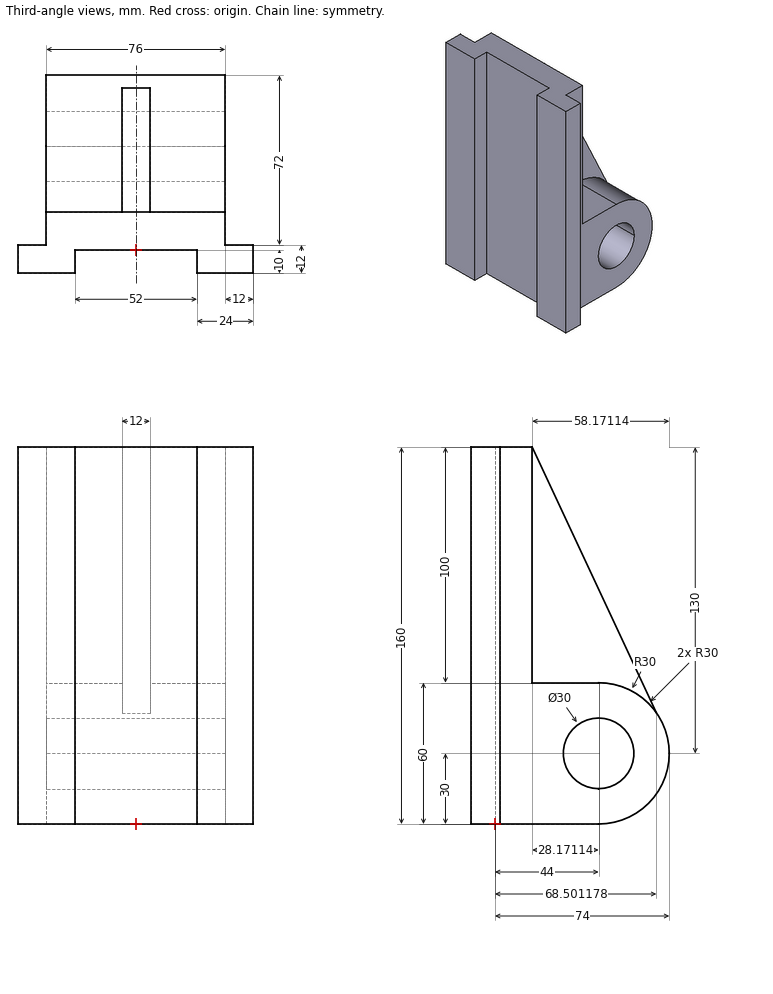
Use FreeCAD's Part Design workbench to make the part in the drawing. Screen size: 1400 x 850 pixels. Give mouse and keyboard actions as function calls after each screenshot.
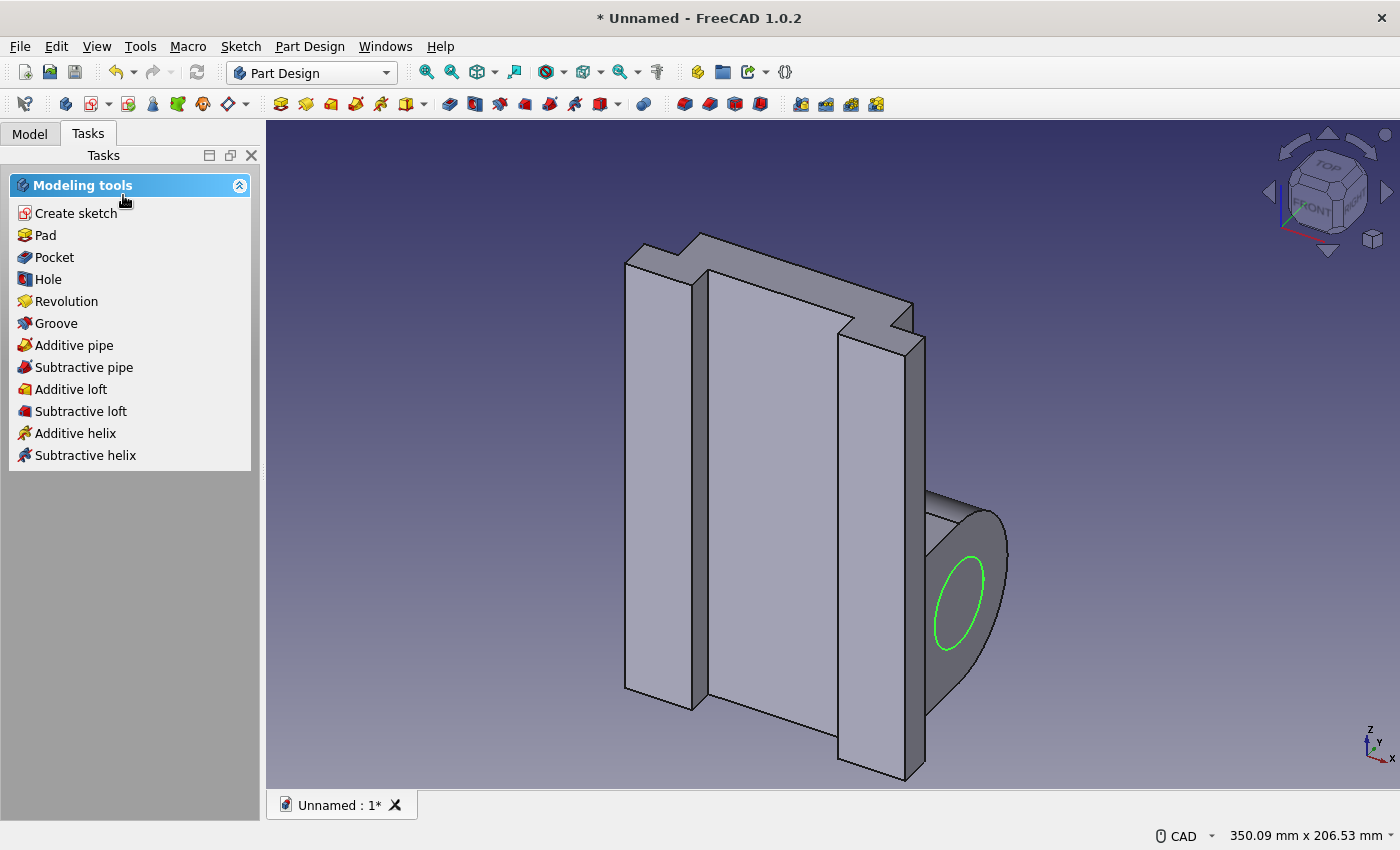
click(450, 104)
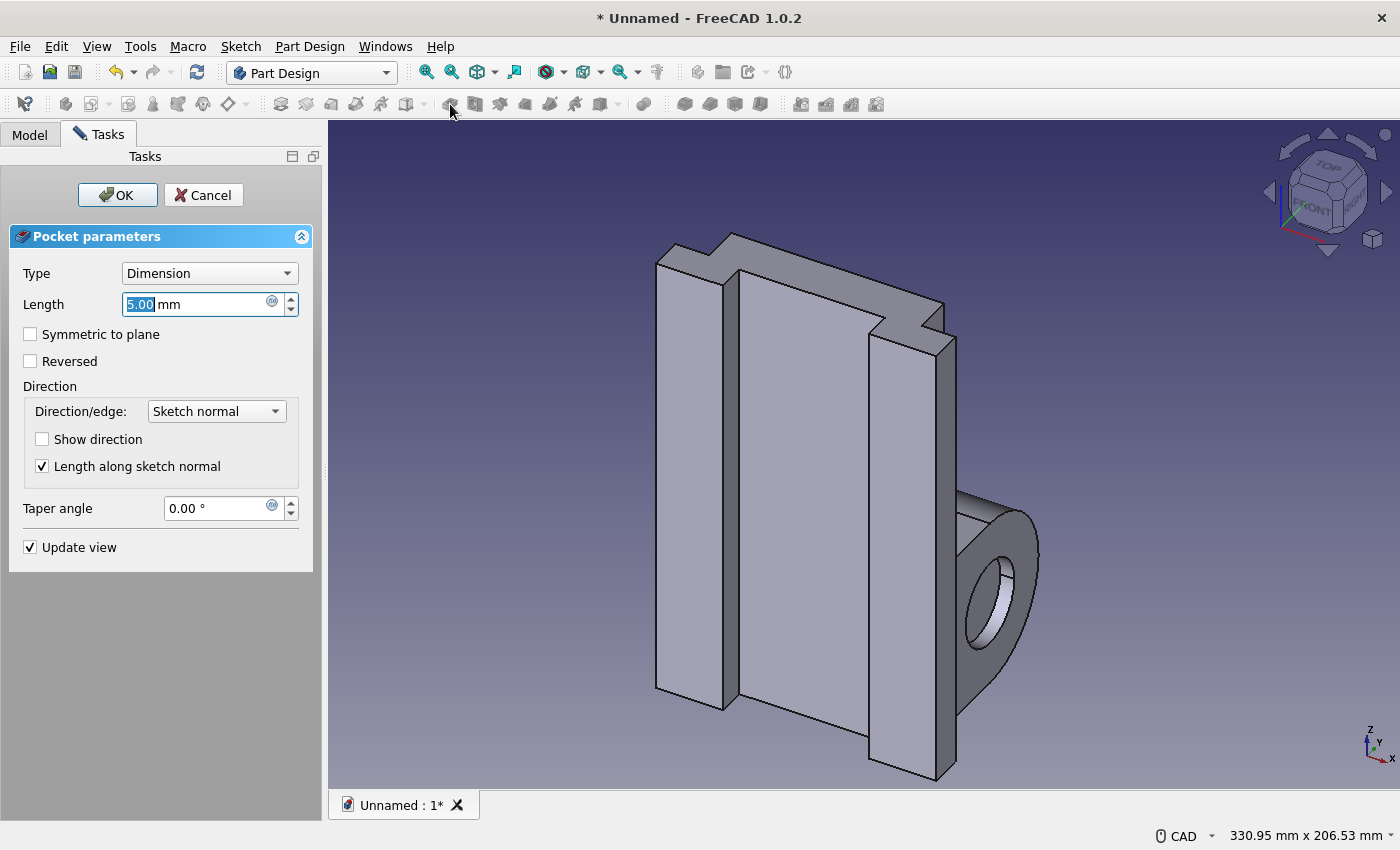
click(210, 274)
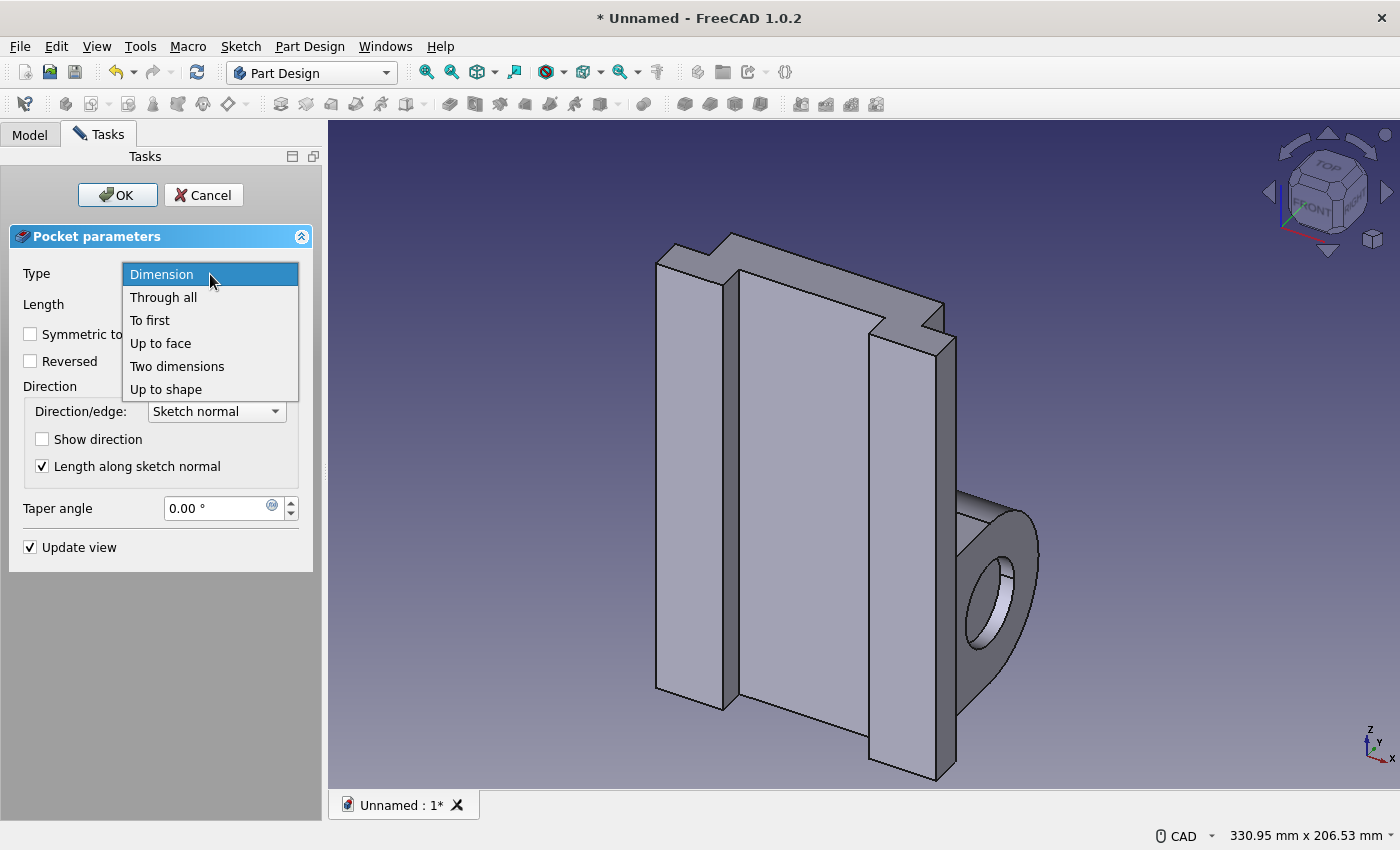
click(208, 298)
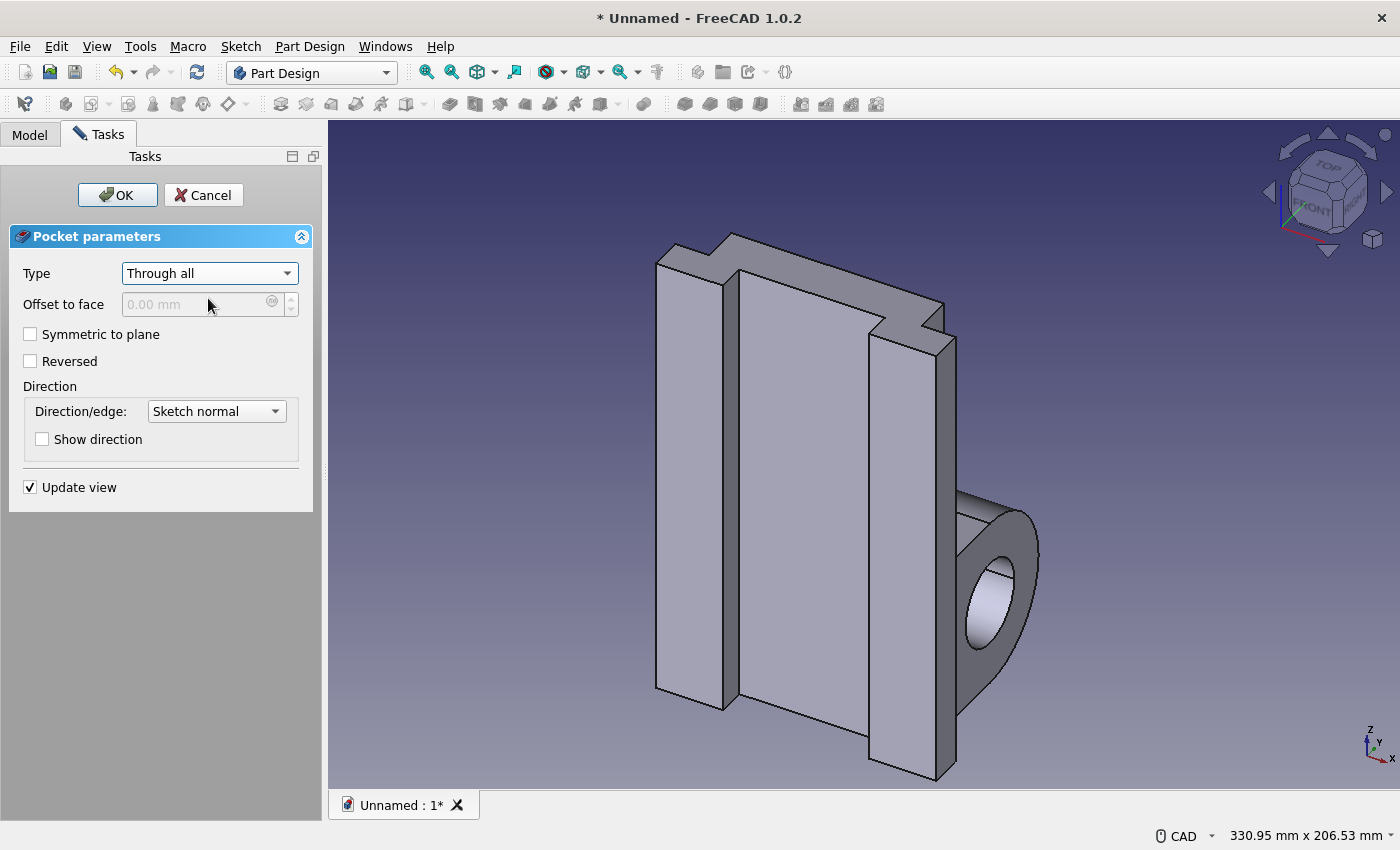
click(118, 195)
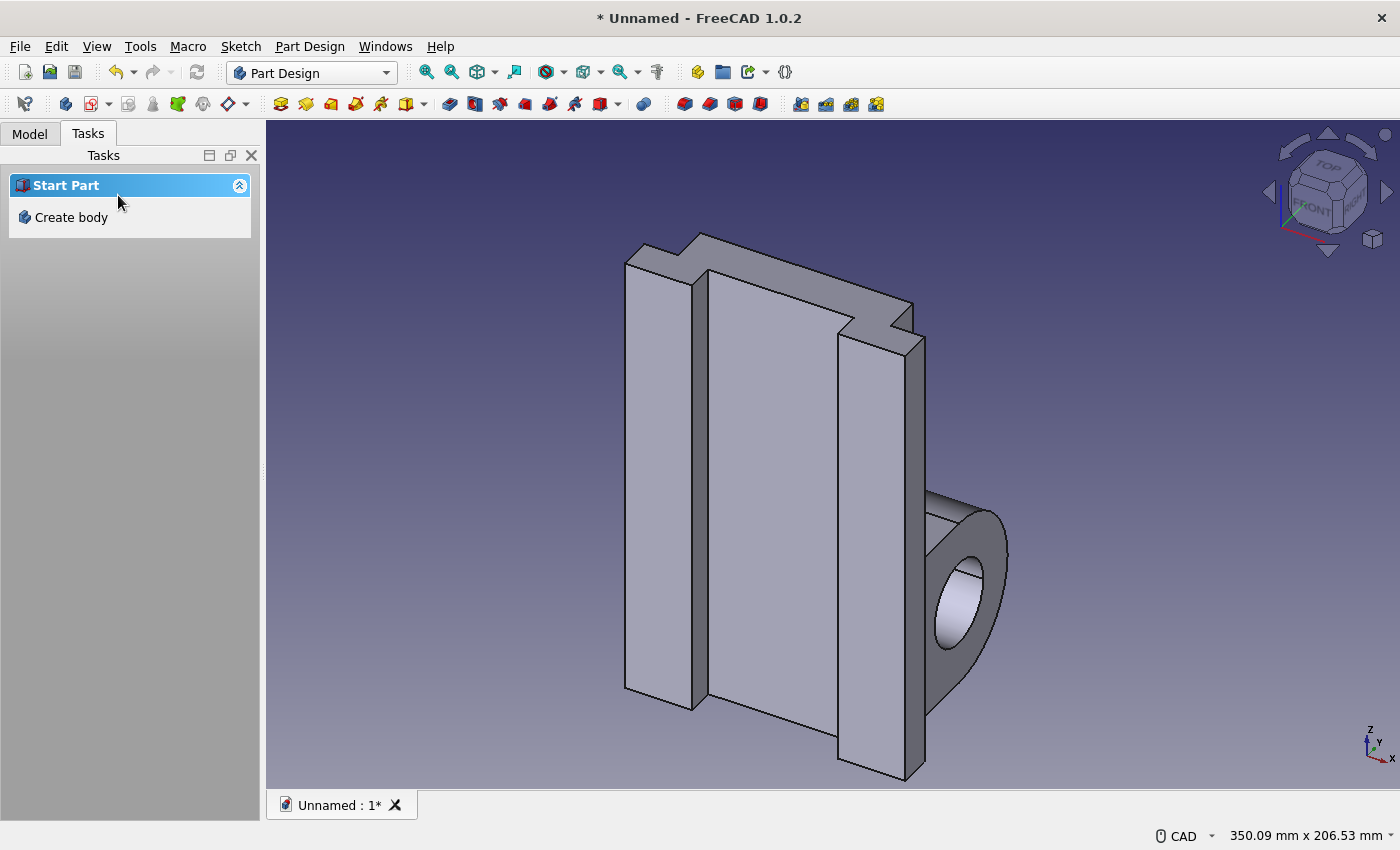
key(0)